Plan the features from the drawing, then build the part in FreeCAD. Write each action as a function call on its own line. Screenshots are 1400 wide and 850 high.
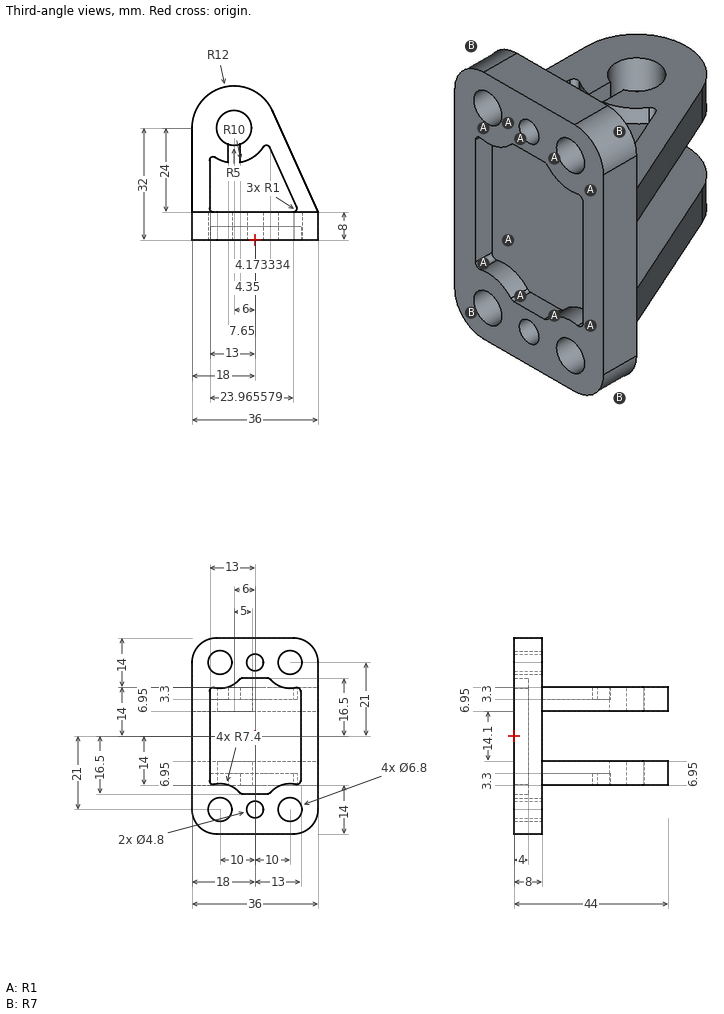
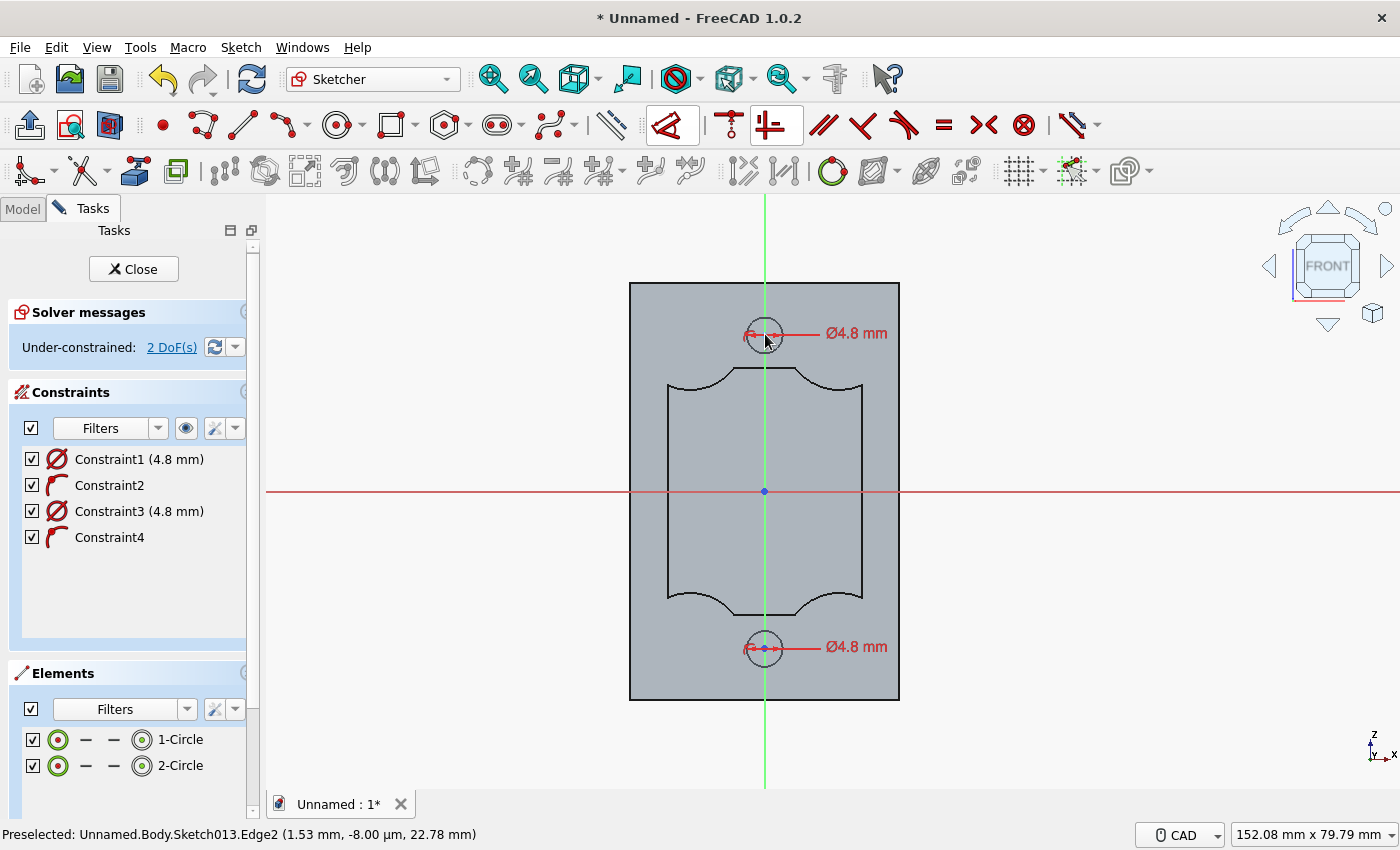
click(765, 649)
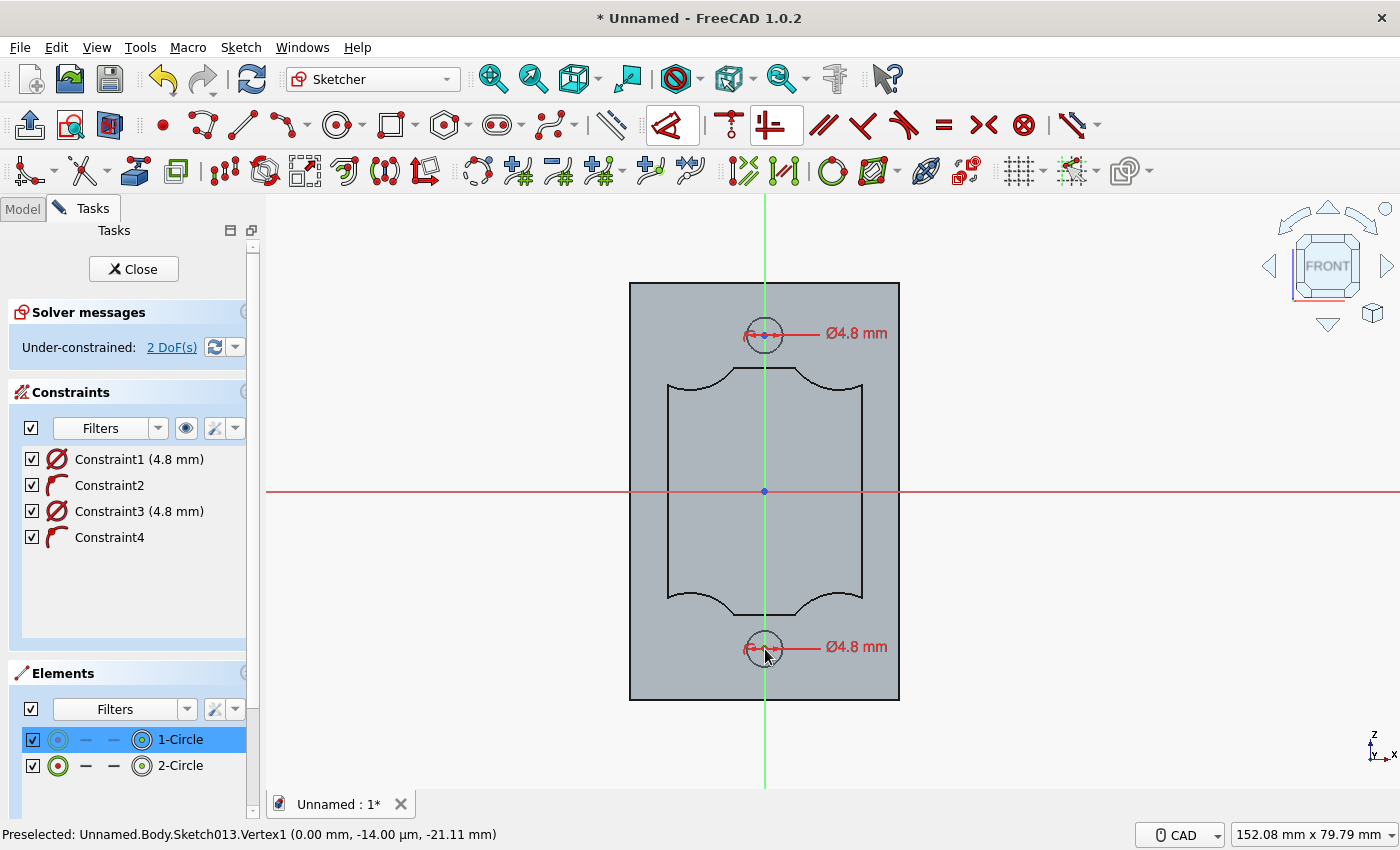
key(i)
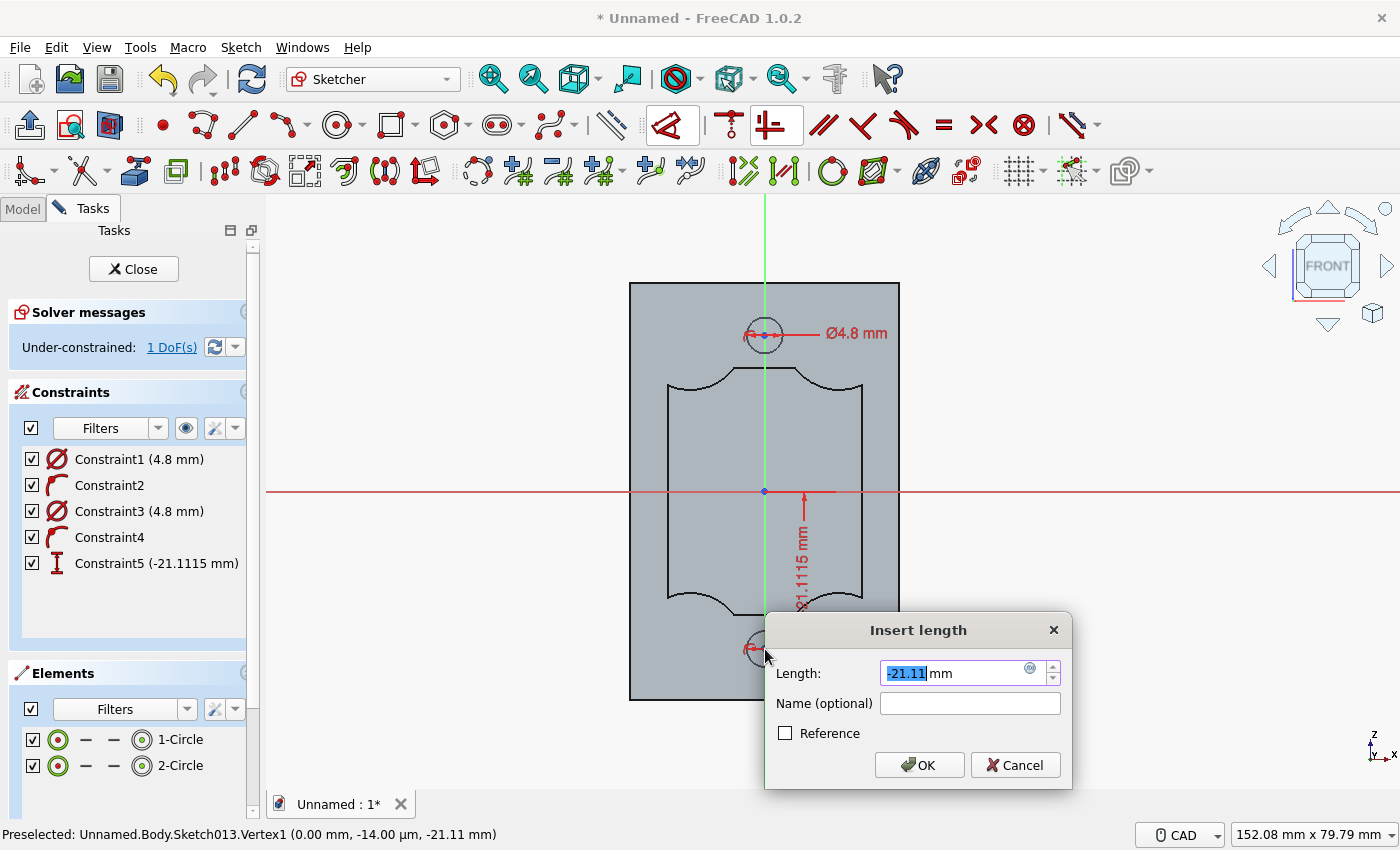
text(-21)
key(Return)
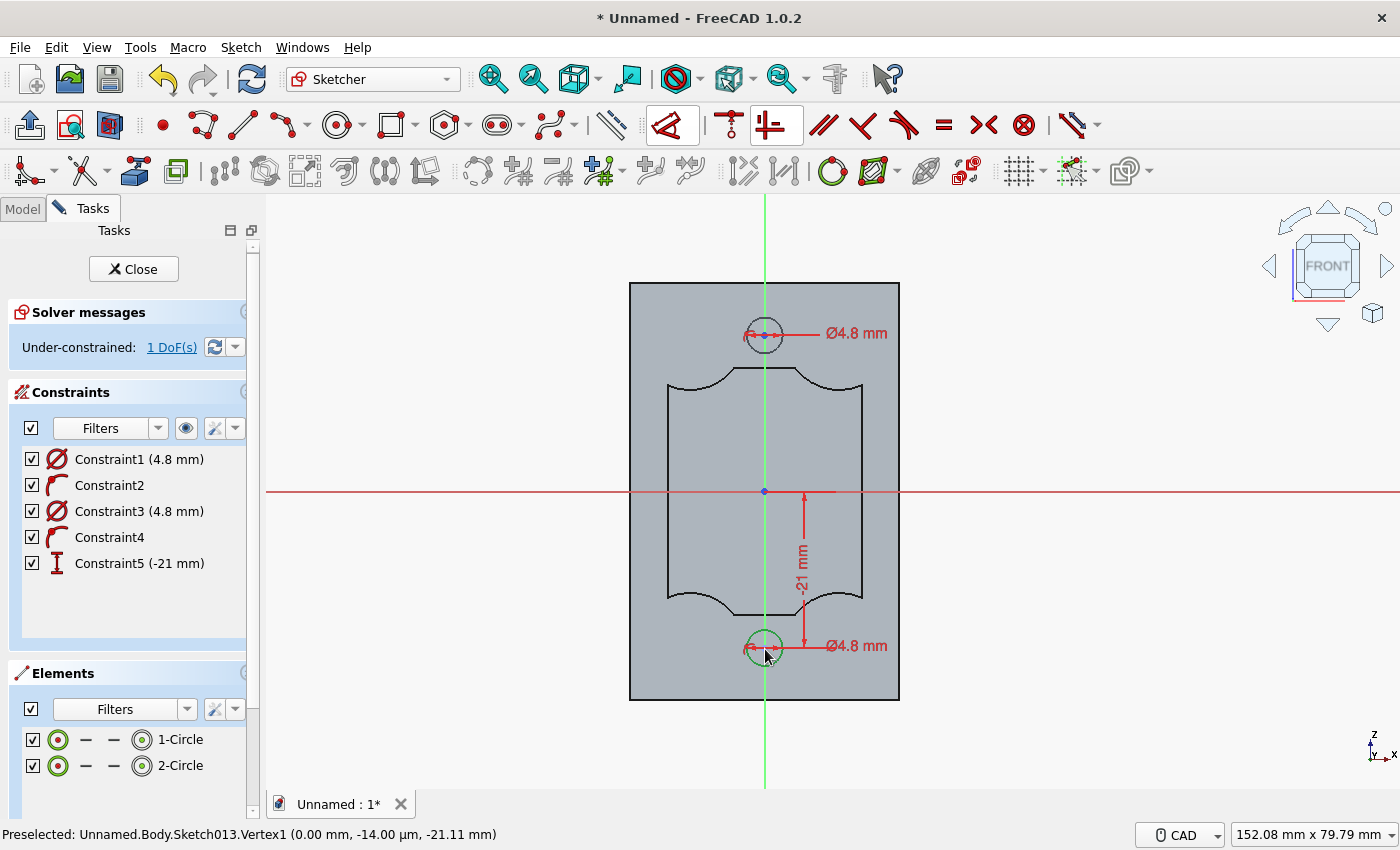
click(765, 335)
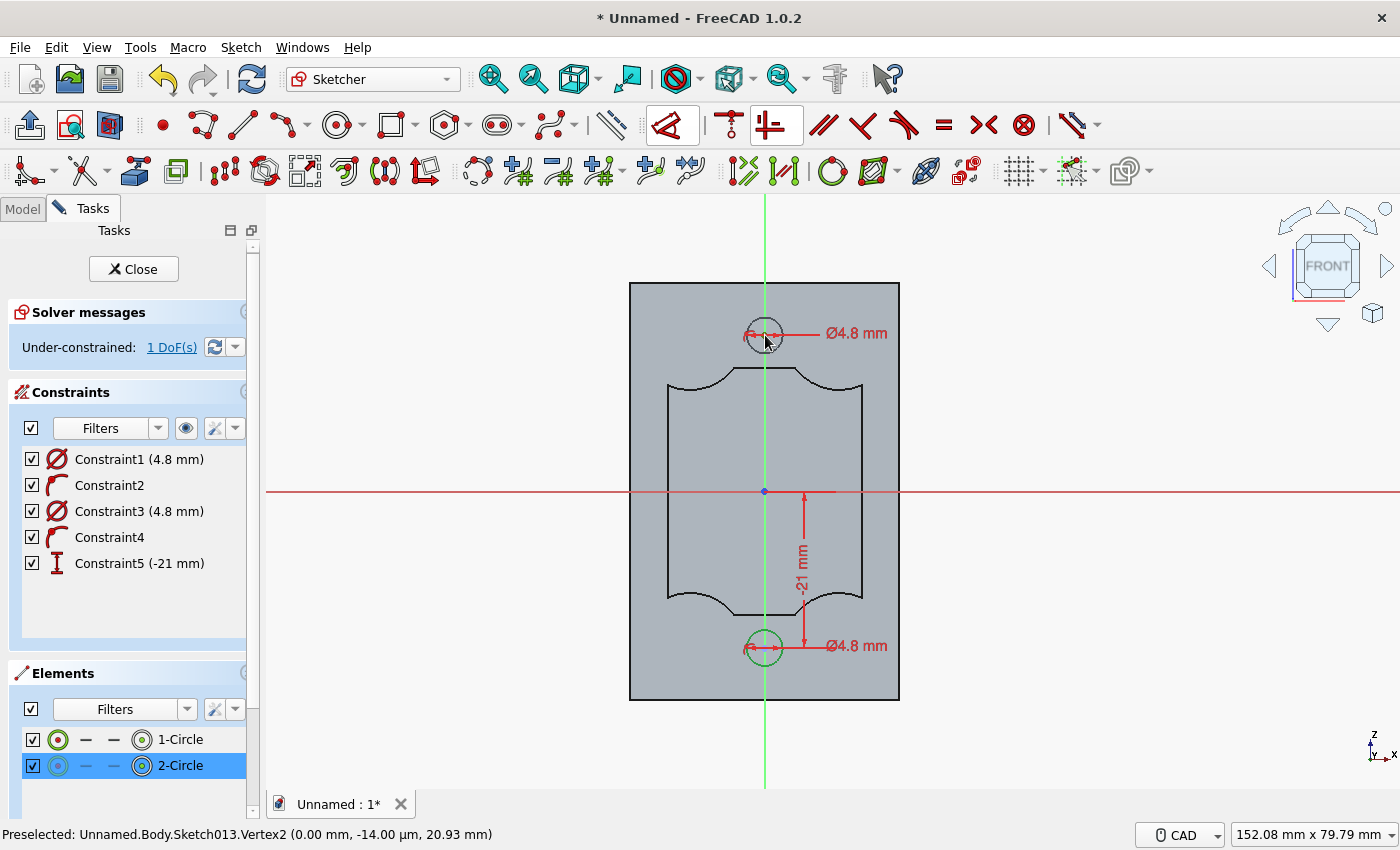
key(i)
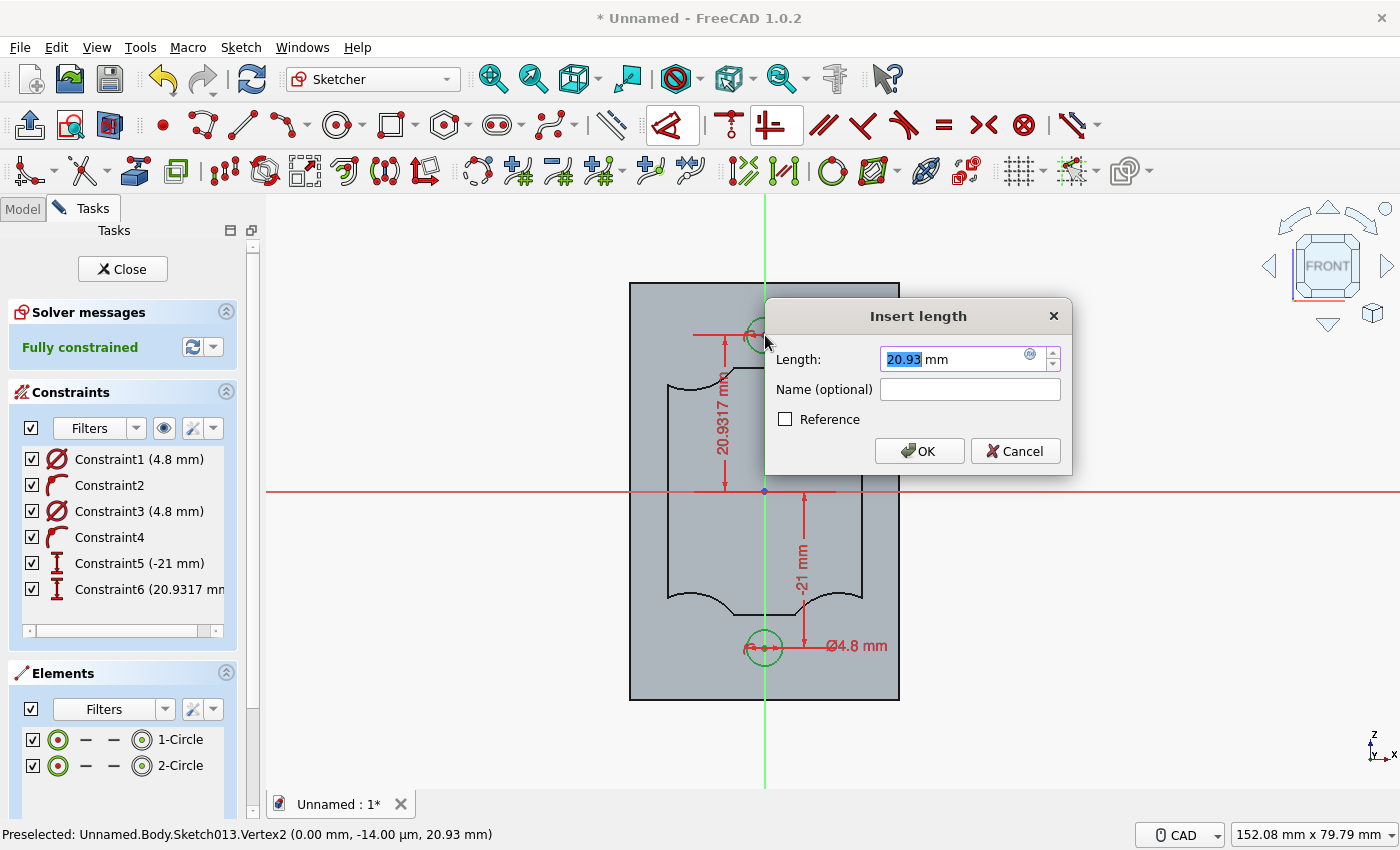
text(21)
key(Return)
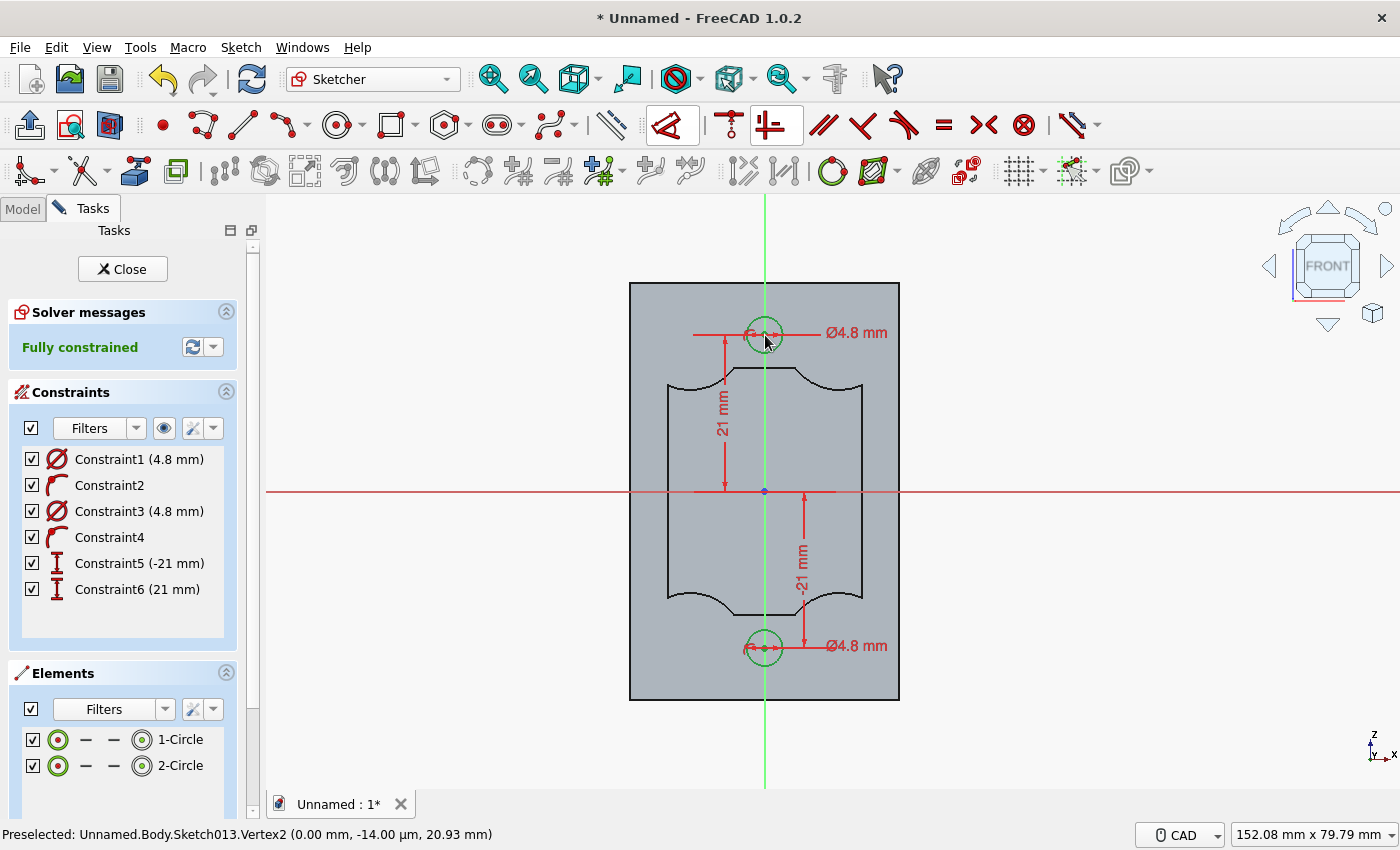
click(123, 269)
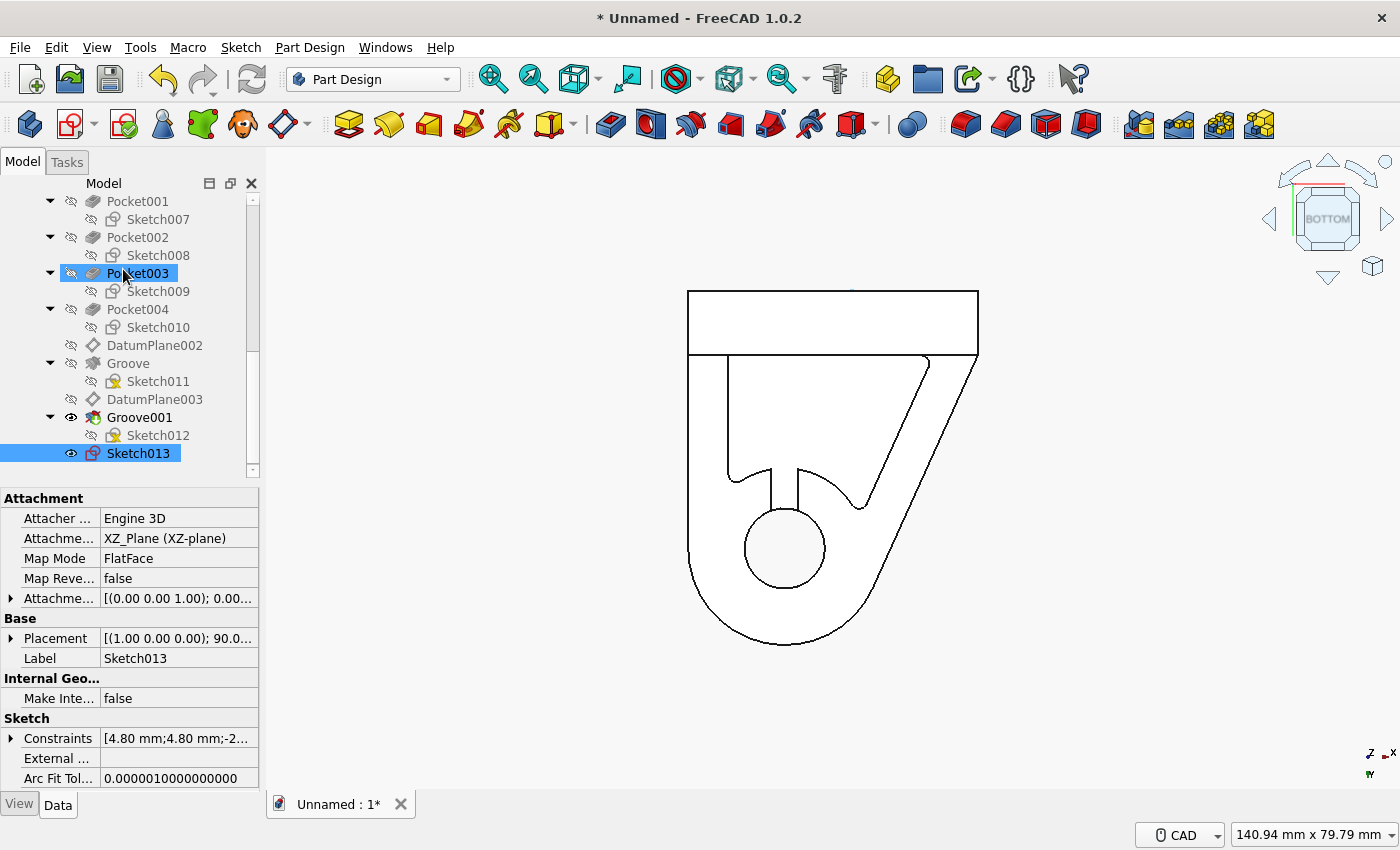
click(612, 124)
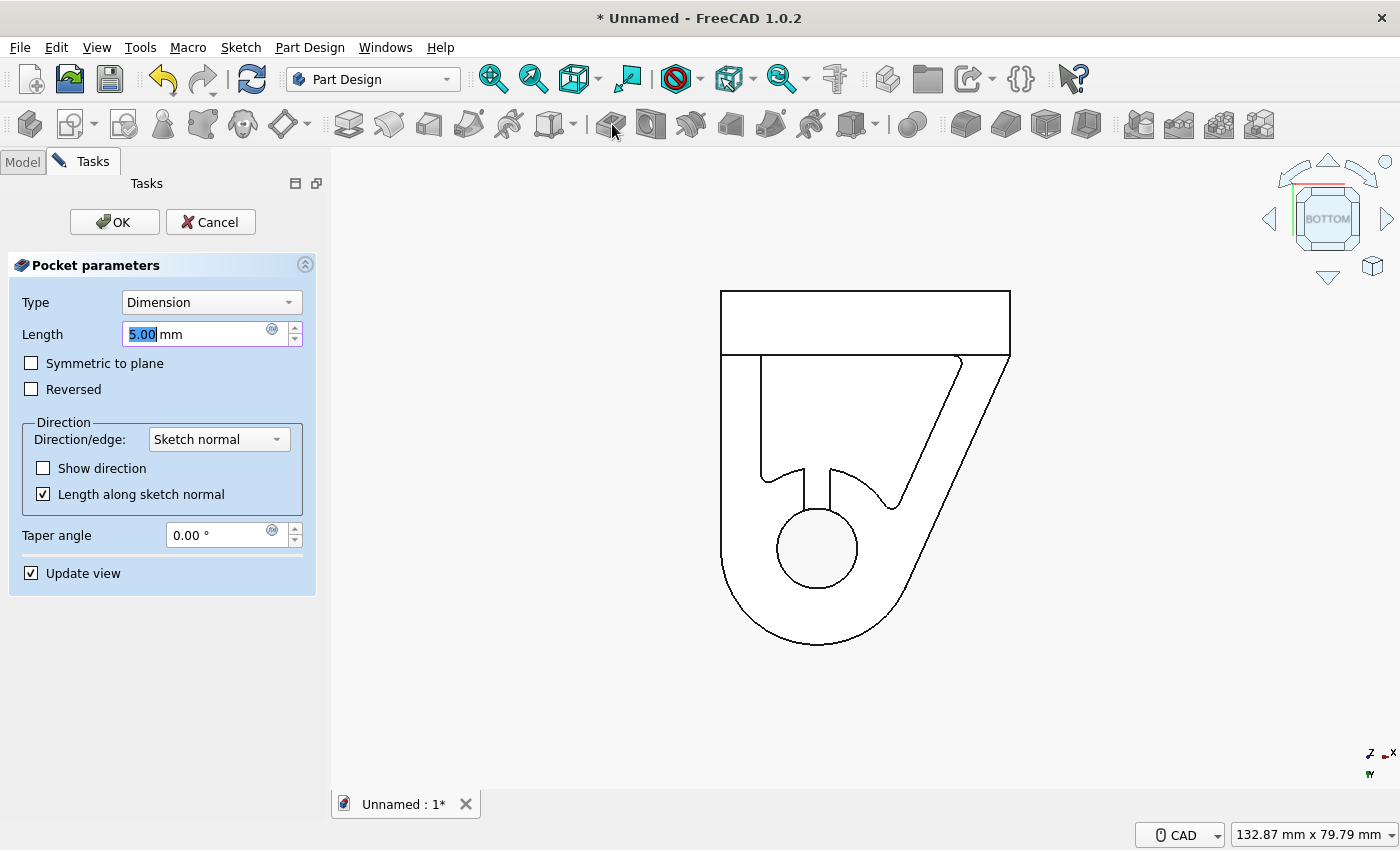
text(44)
key(Tab)